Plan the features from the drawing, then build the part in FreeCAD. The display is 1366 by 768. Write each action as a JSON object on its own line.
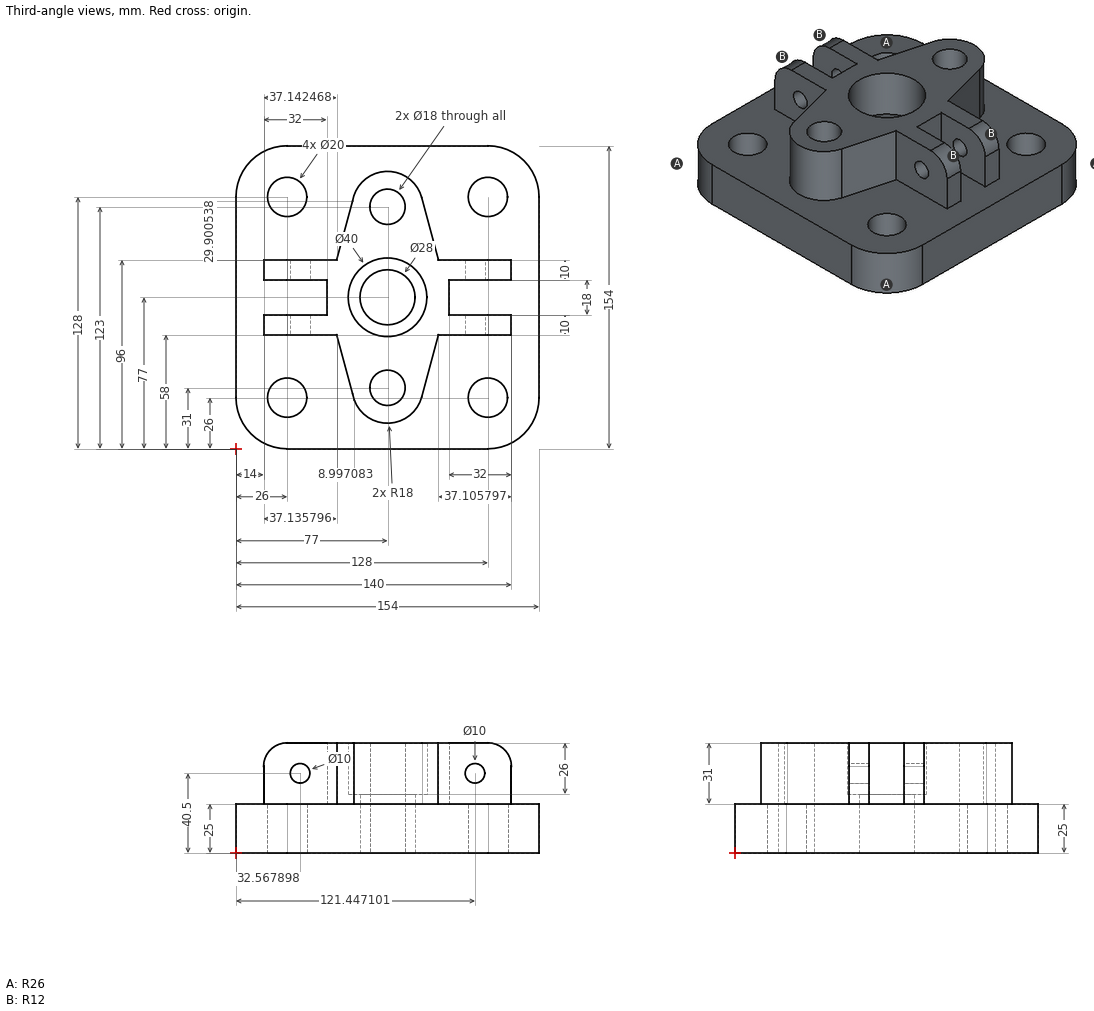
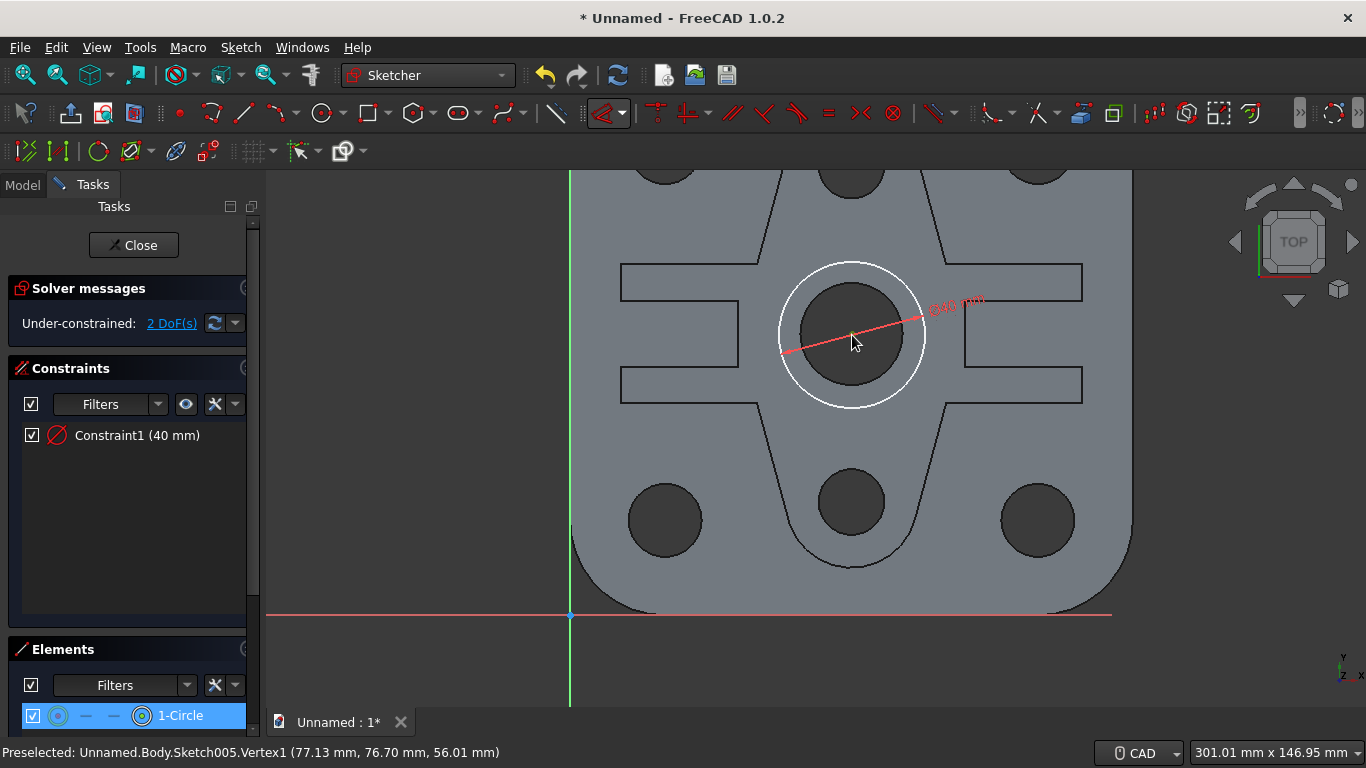
{"action": "left_click", "coordinate": [624, 114]}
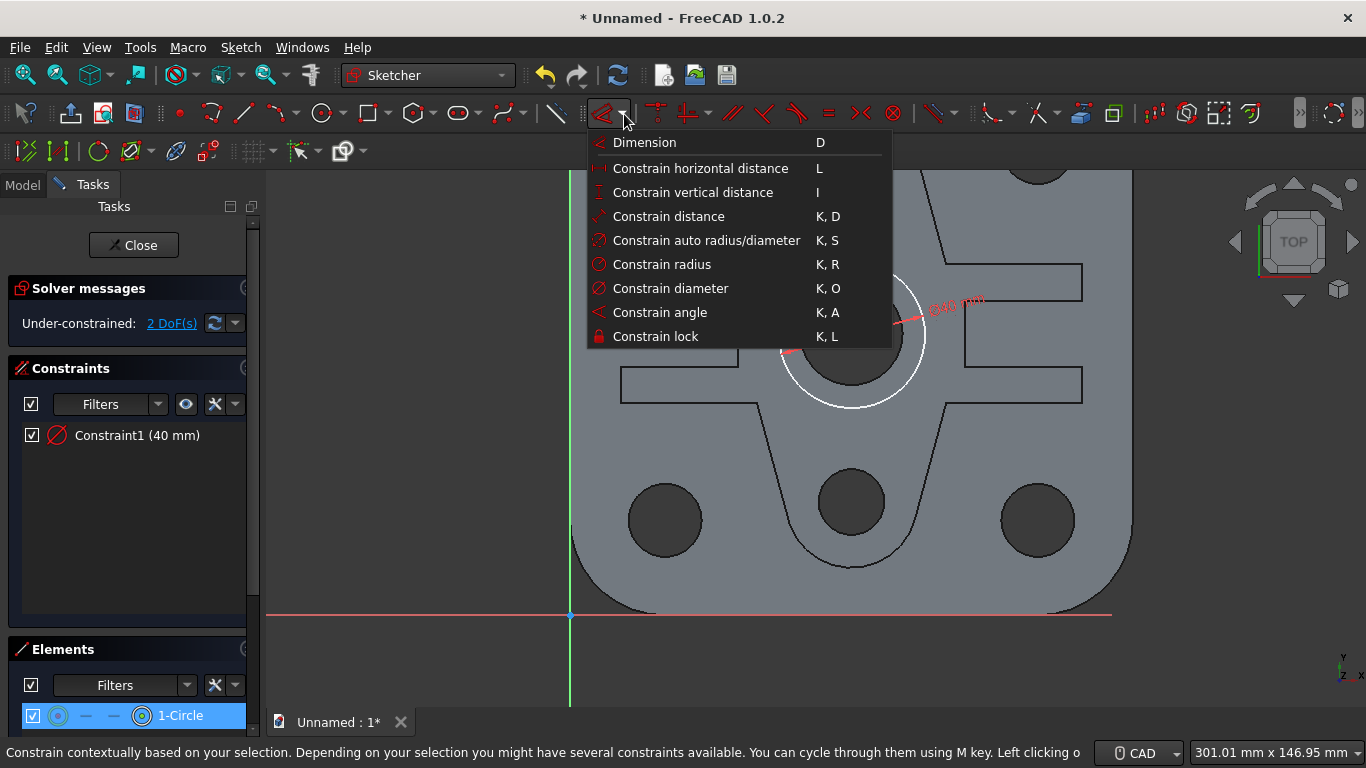
{"action": "left_click", "coordinate": [740, 168]}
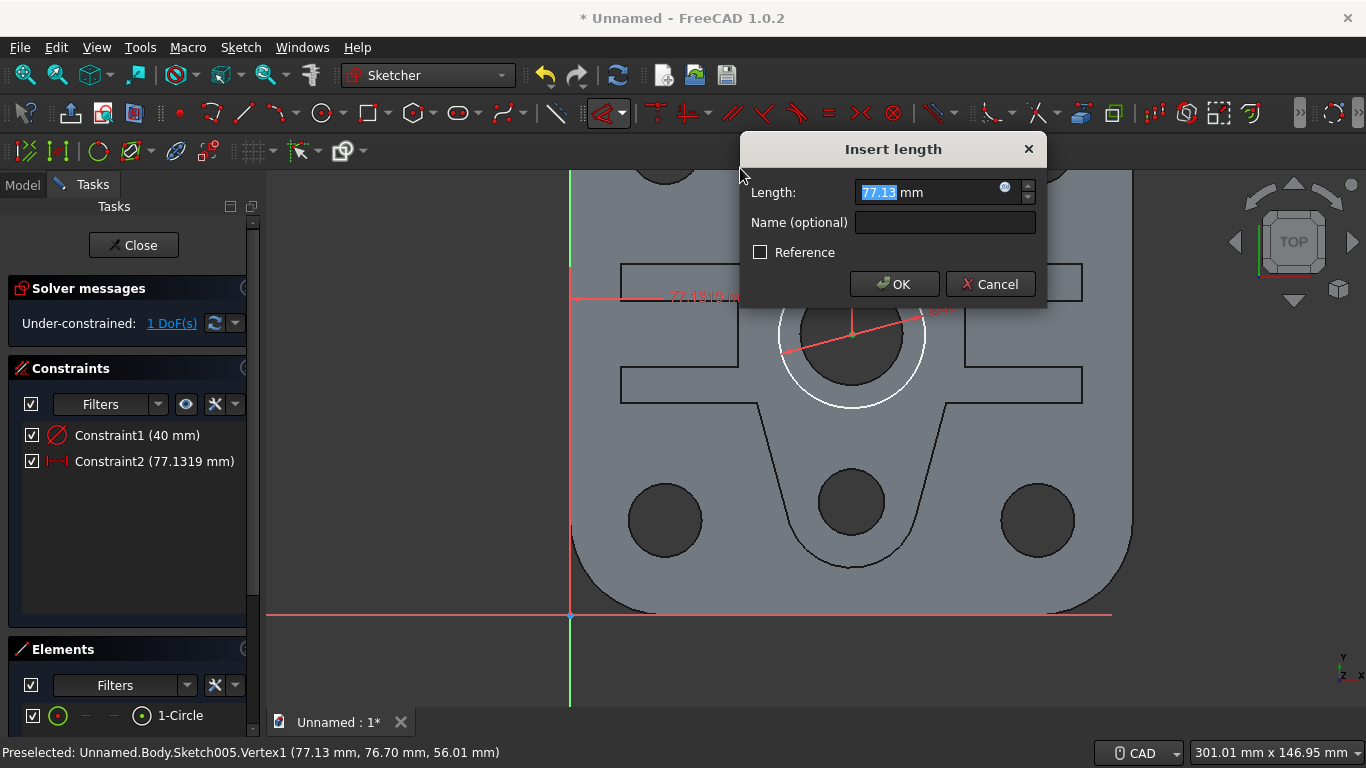
{"action": "type", "text": "77"}
{"action": "key", "text": "Return"}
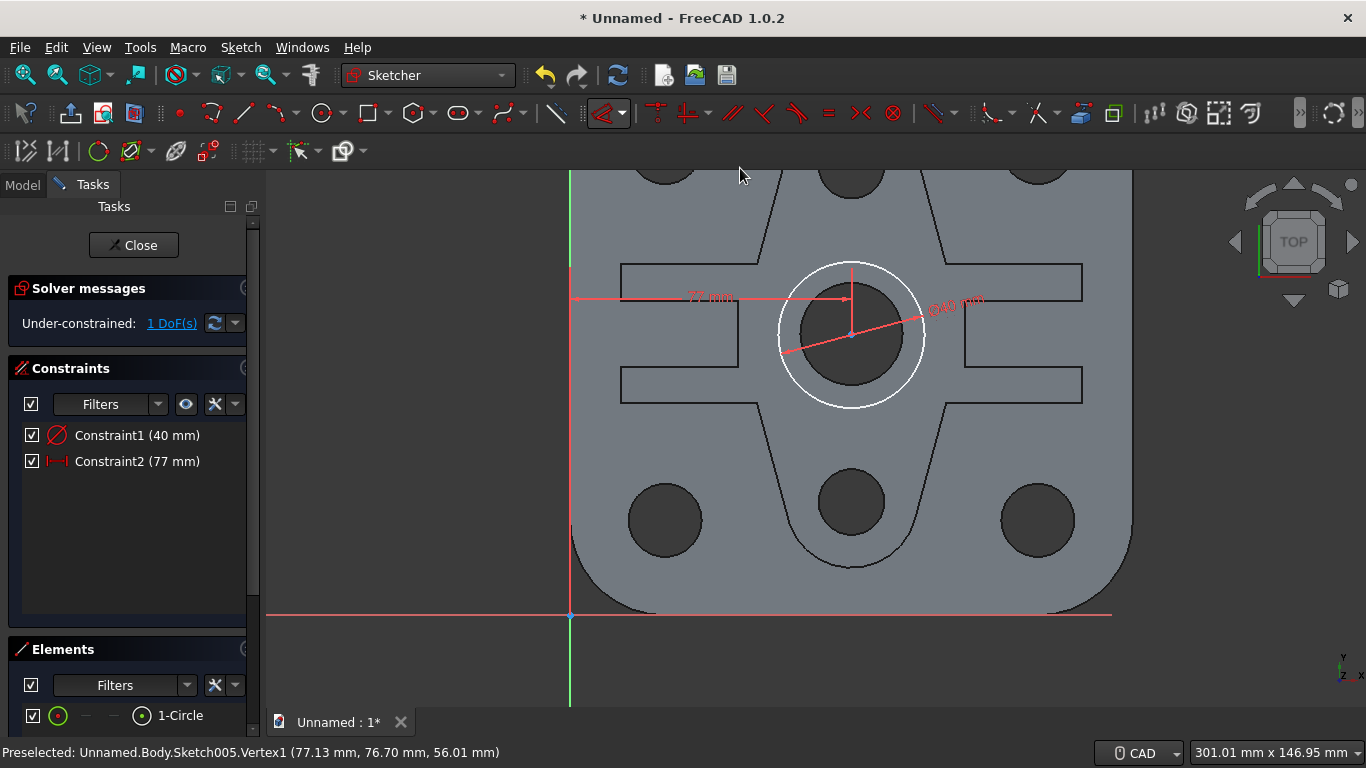
{"action": "left_click", "coordinate": [852, 335]}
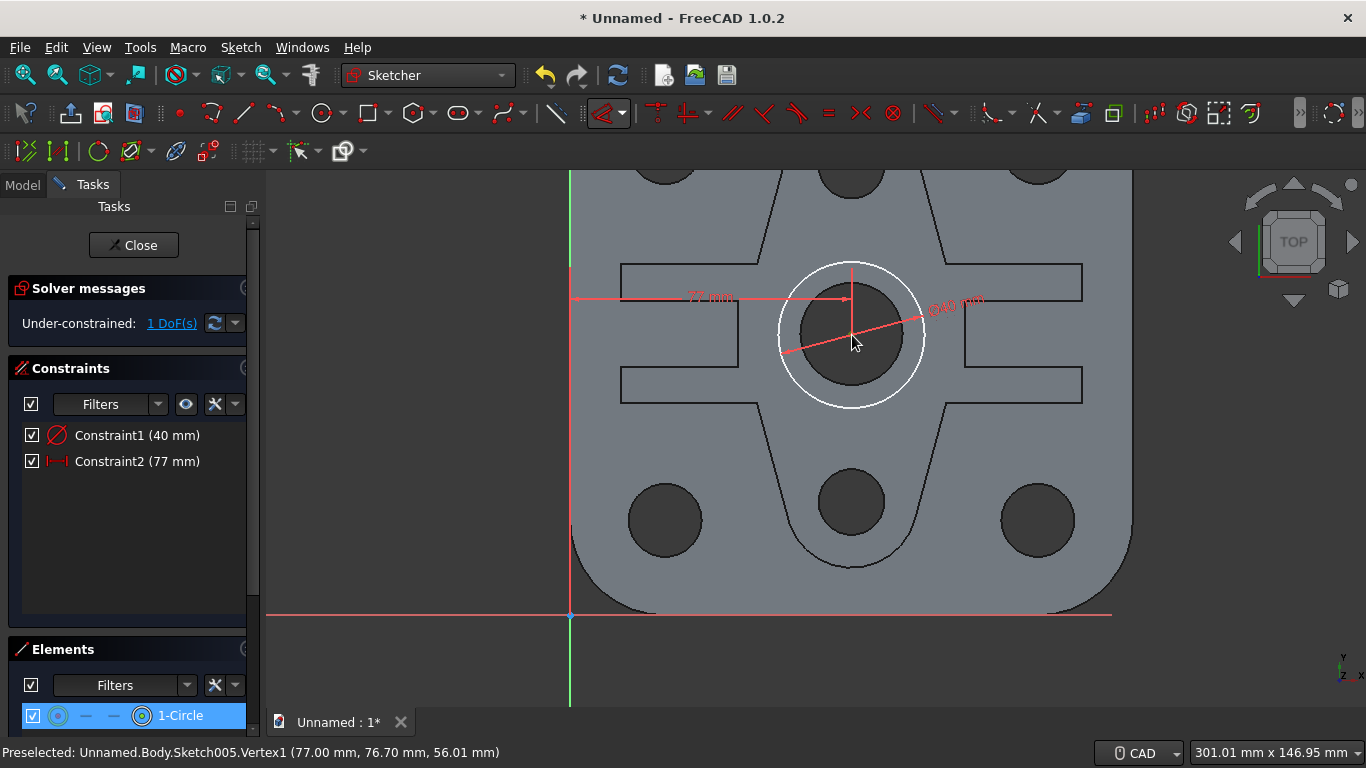
{"action": "key", "text": "i"}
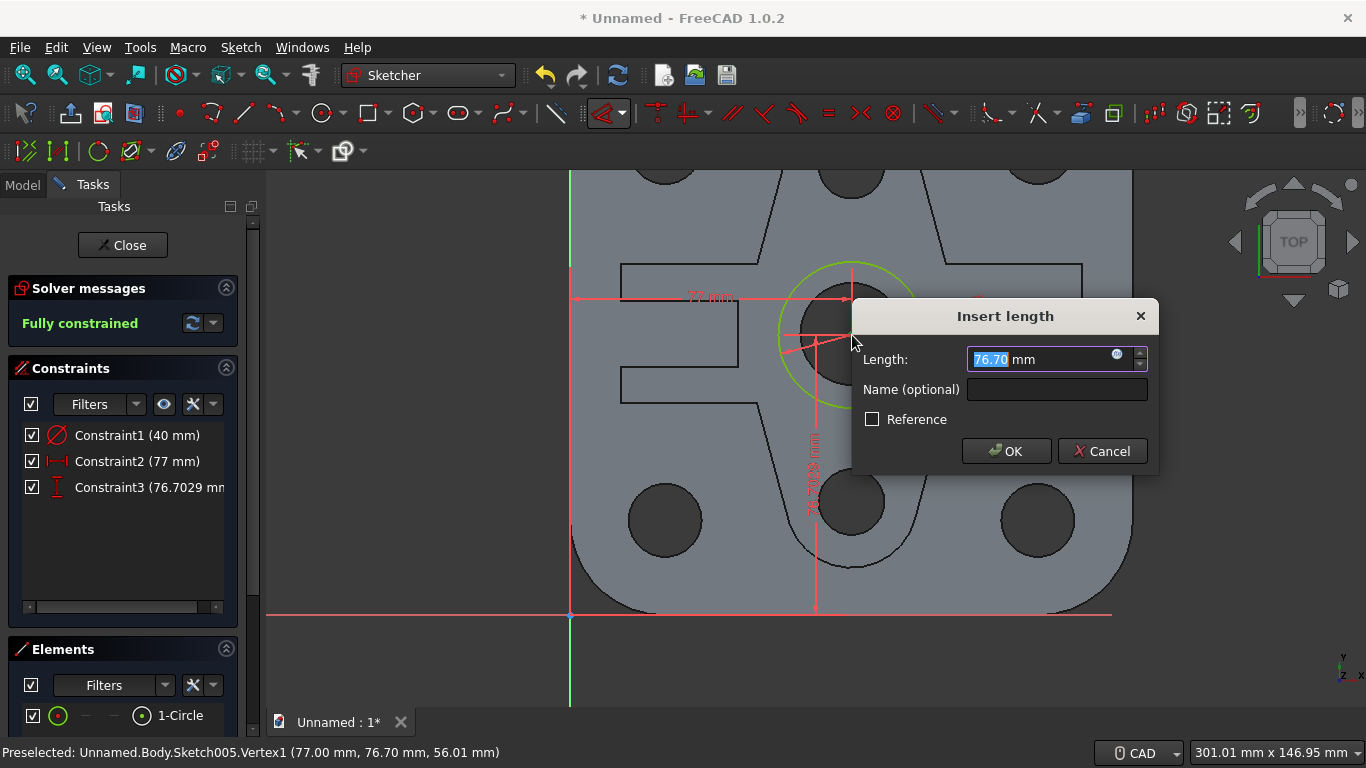
{"action": "type", "text": "77"}
{"action": "key", "text": "Return"}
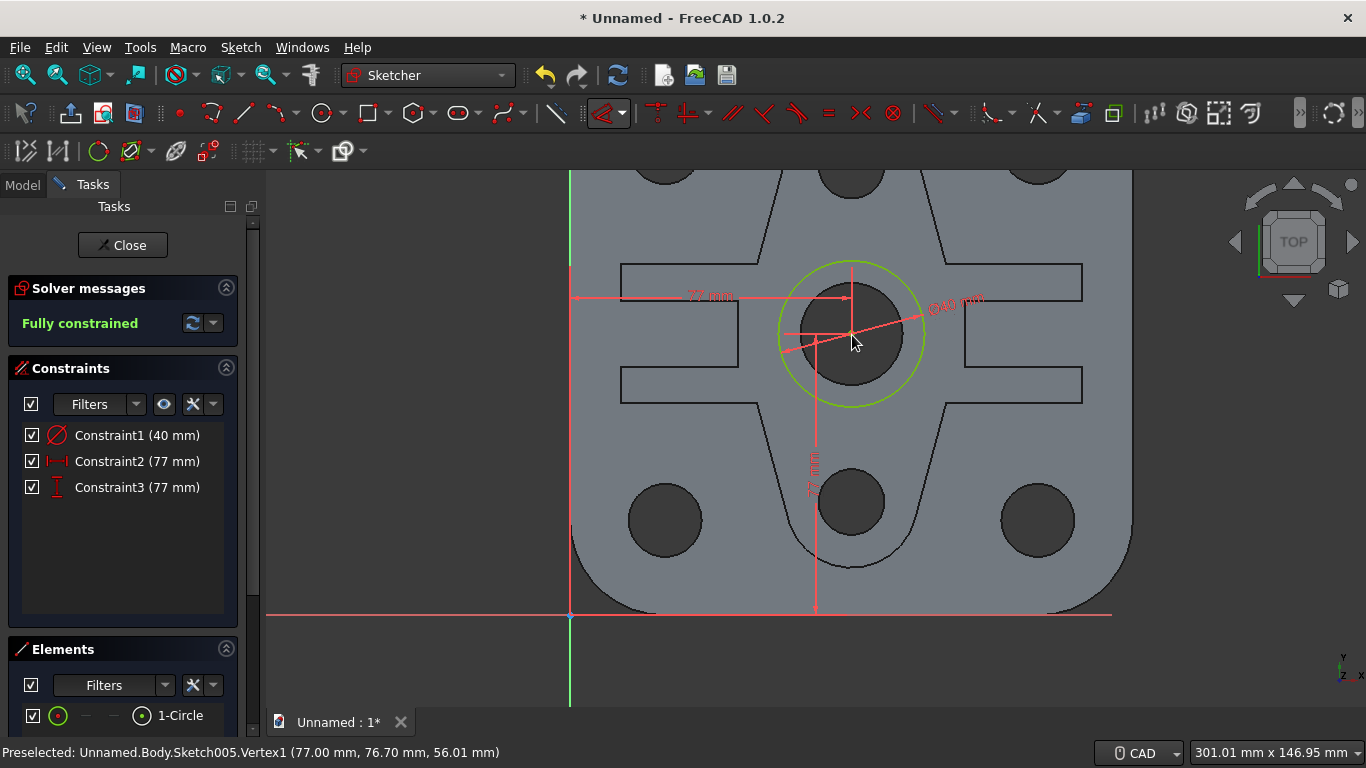
{"action": "left_click", "coordinate": [123, 245]}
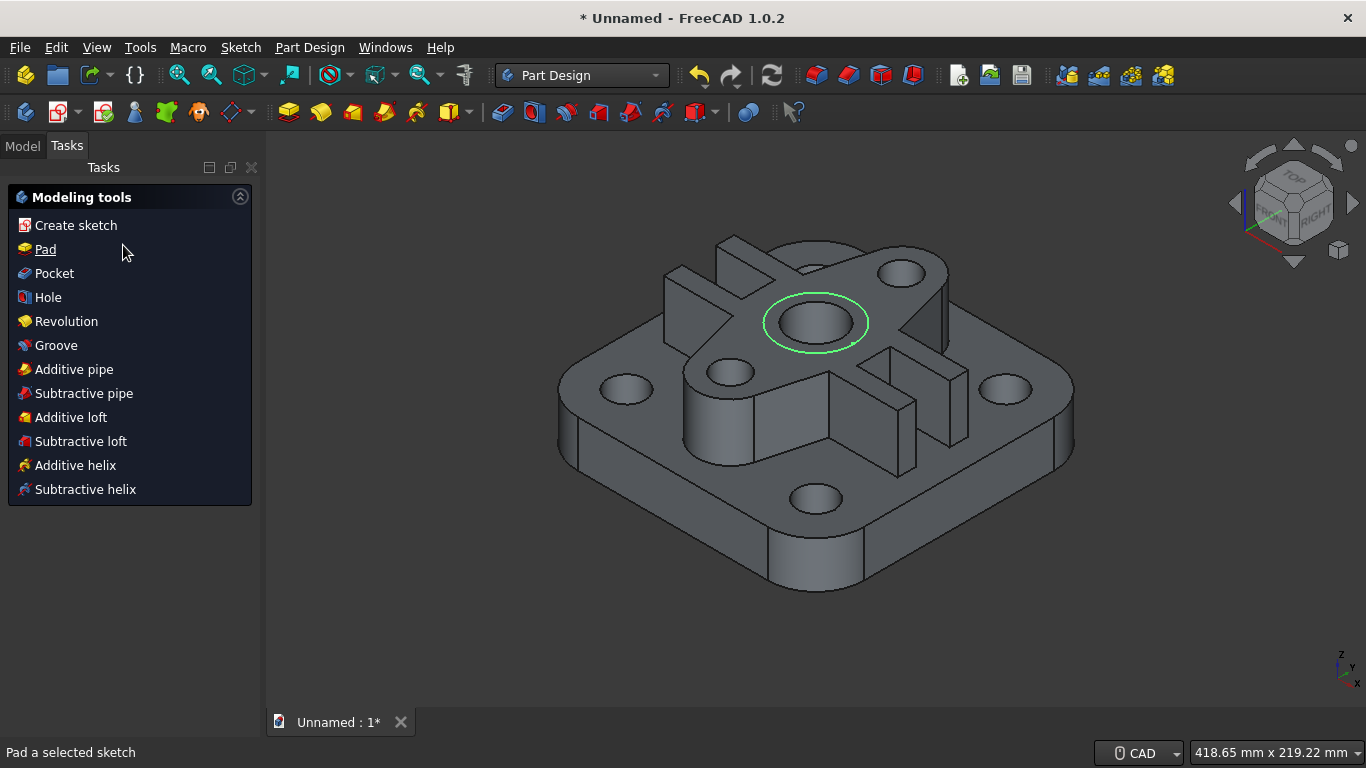
{"action": "left_click", "coordinate": [504, 112]}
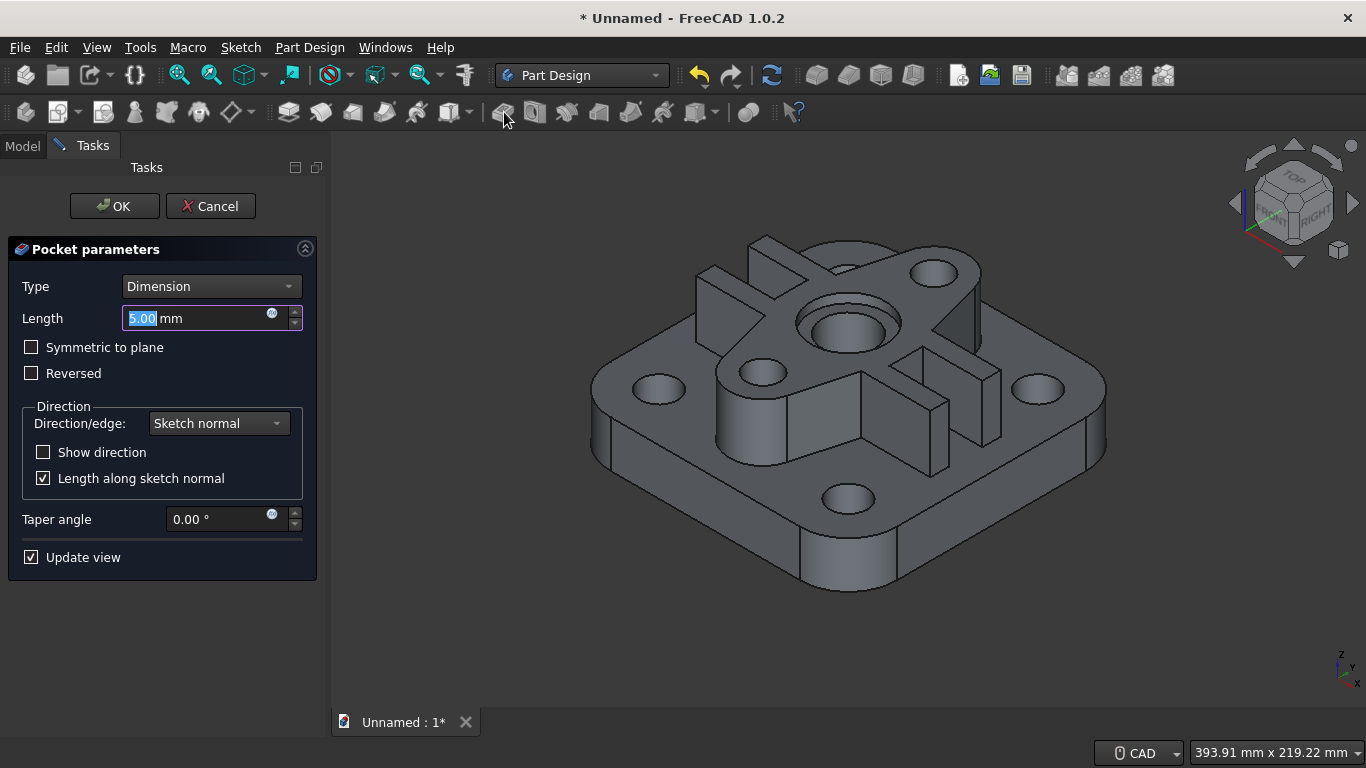
{"action": "type", "text": "26"}
{"action": "key", "text": "Tab"}